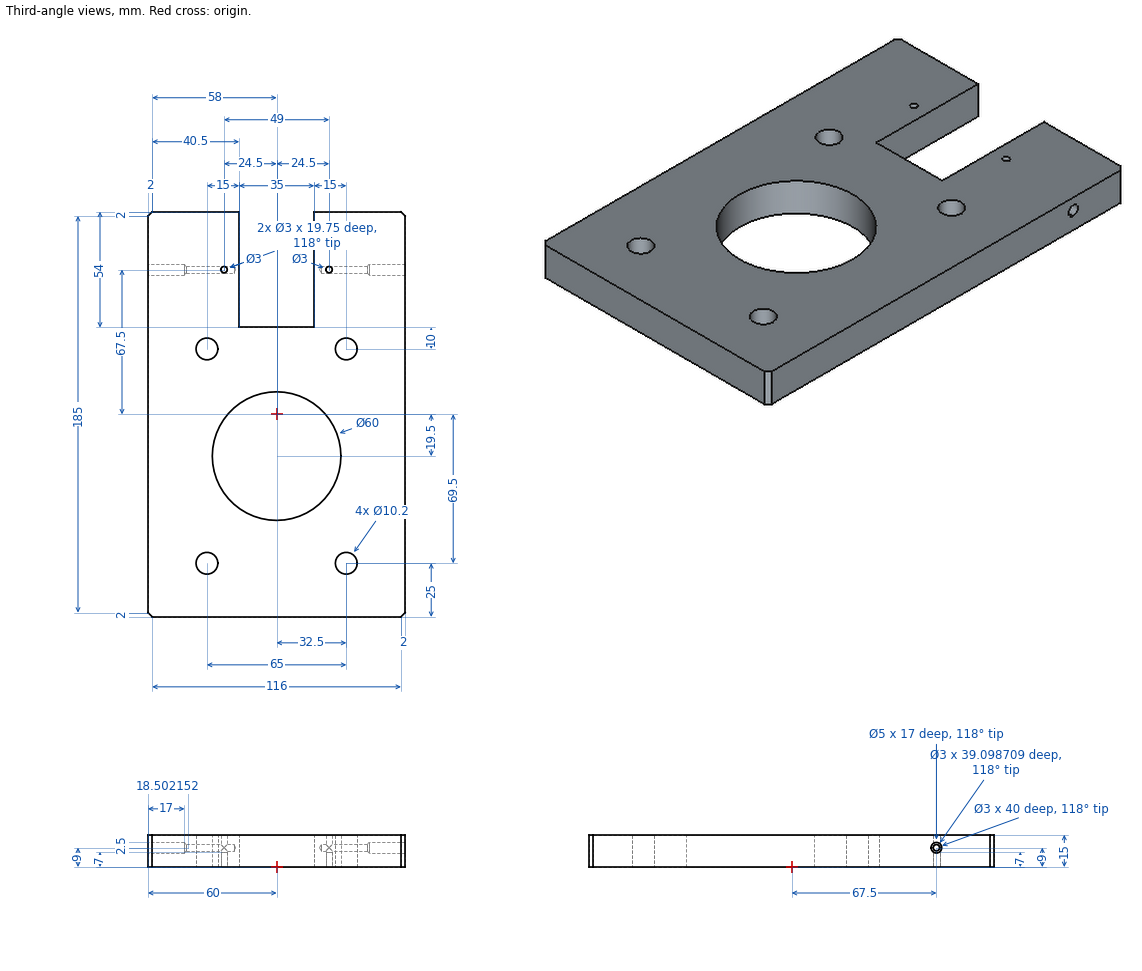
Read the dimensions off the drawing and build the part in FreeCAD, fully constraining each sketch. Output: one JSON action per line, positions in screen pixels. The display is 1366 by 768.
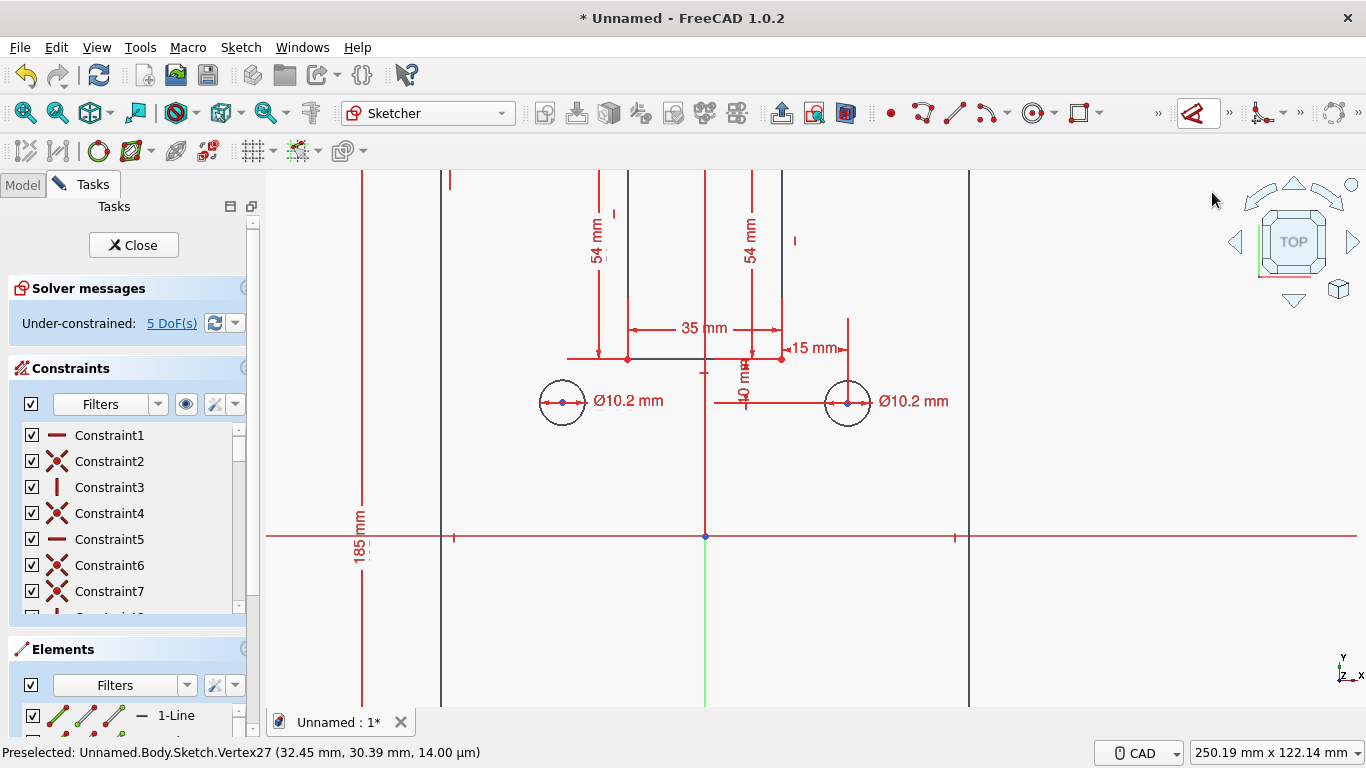
{"action": "left_click", "coordinate": [628, 359]}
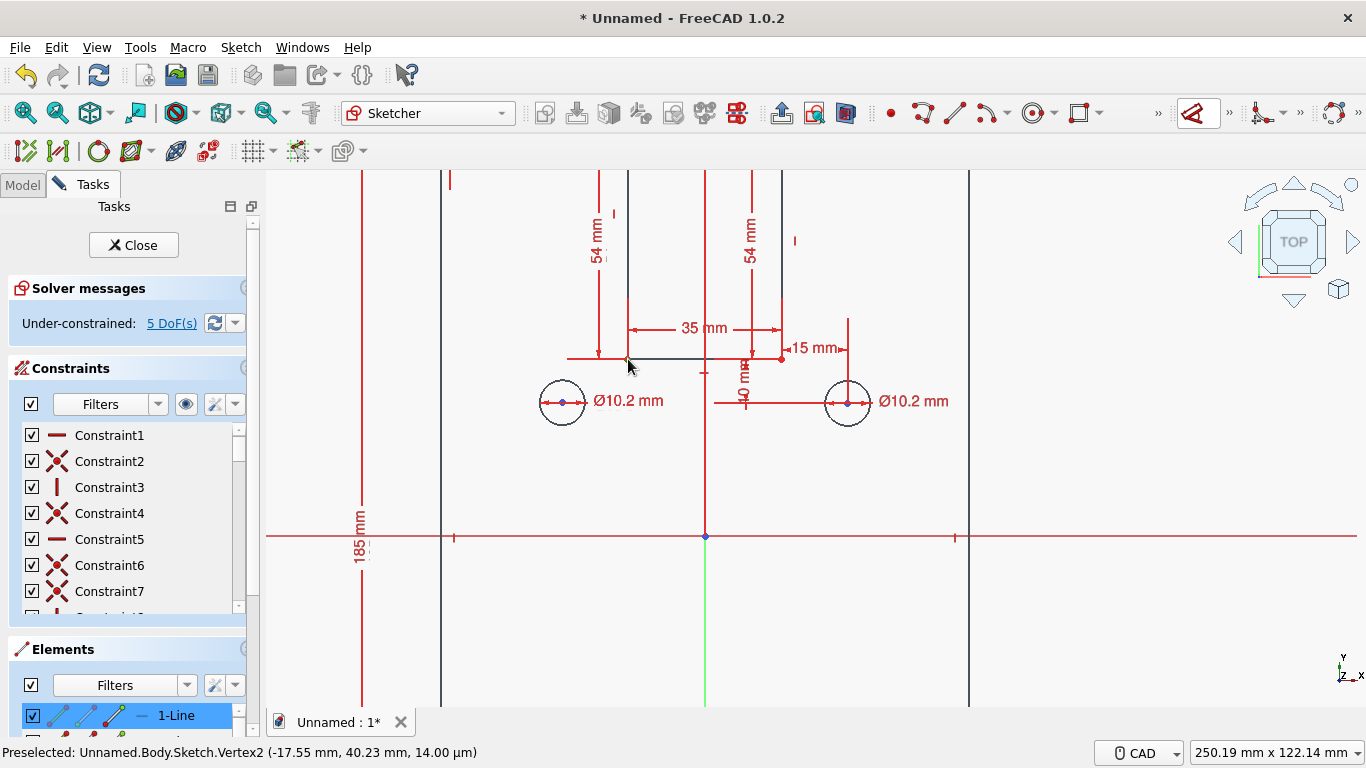
{"action": "left_click", "coordinate": [562, 403]}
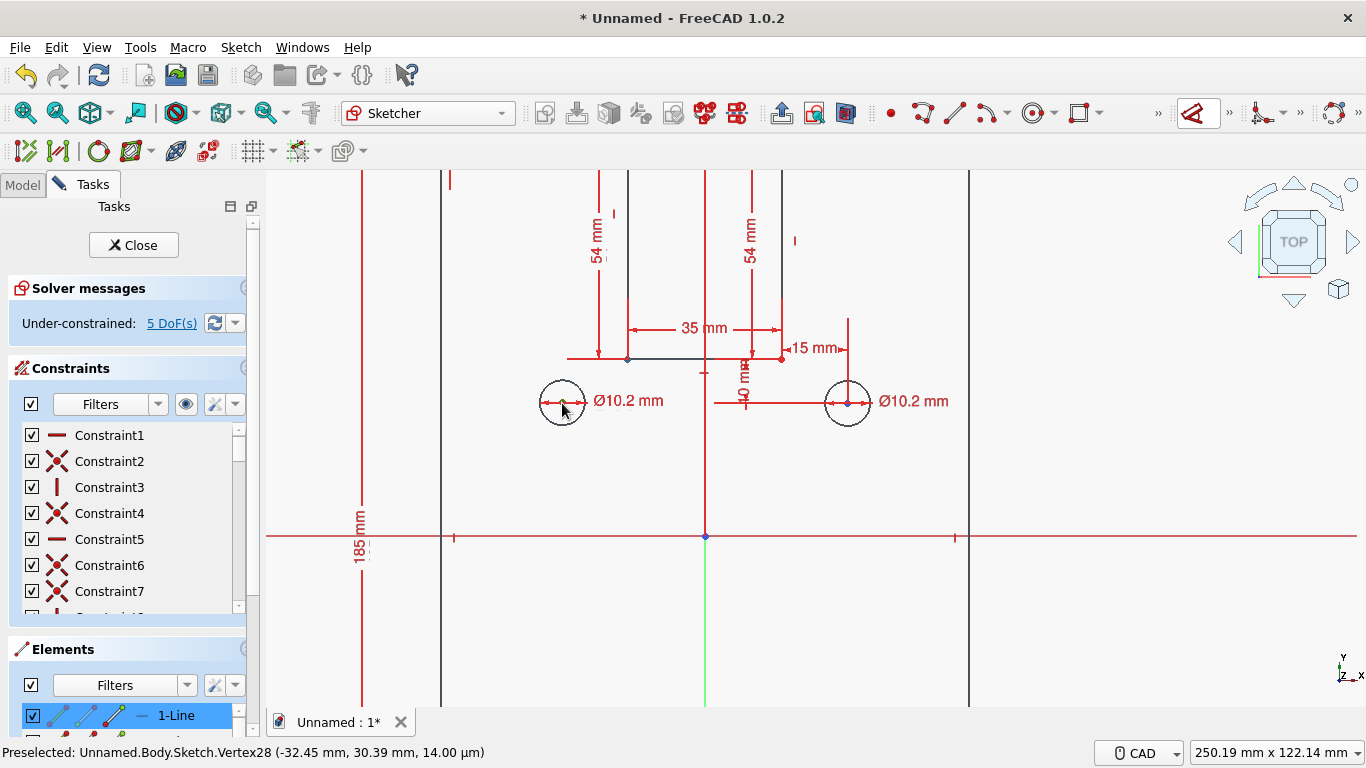
{"action": "key", "text": "l"}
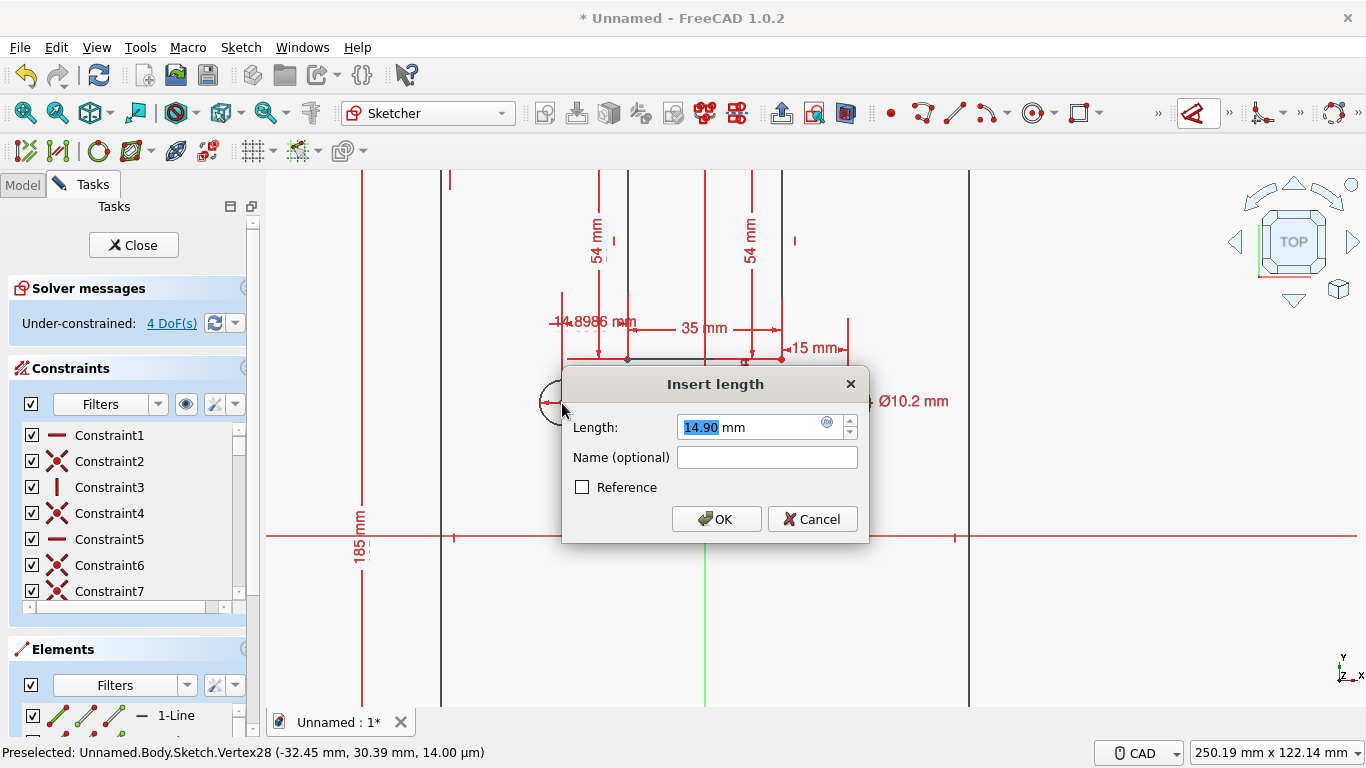
{"action": "type", "text": "15"}
{"action": "key", "text": "Return"}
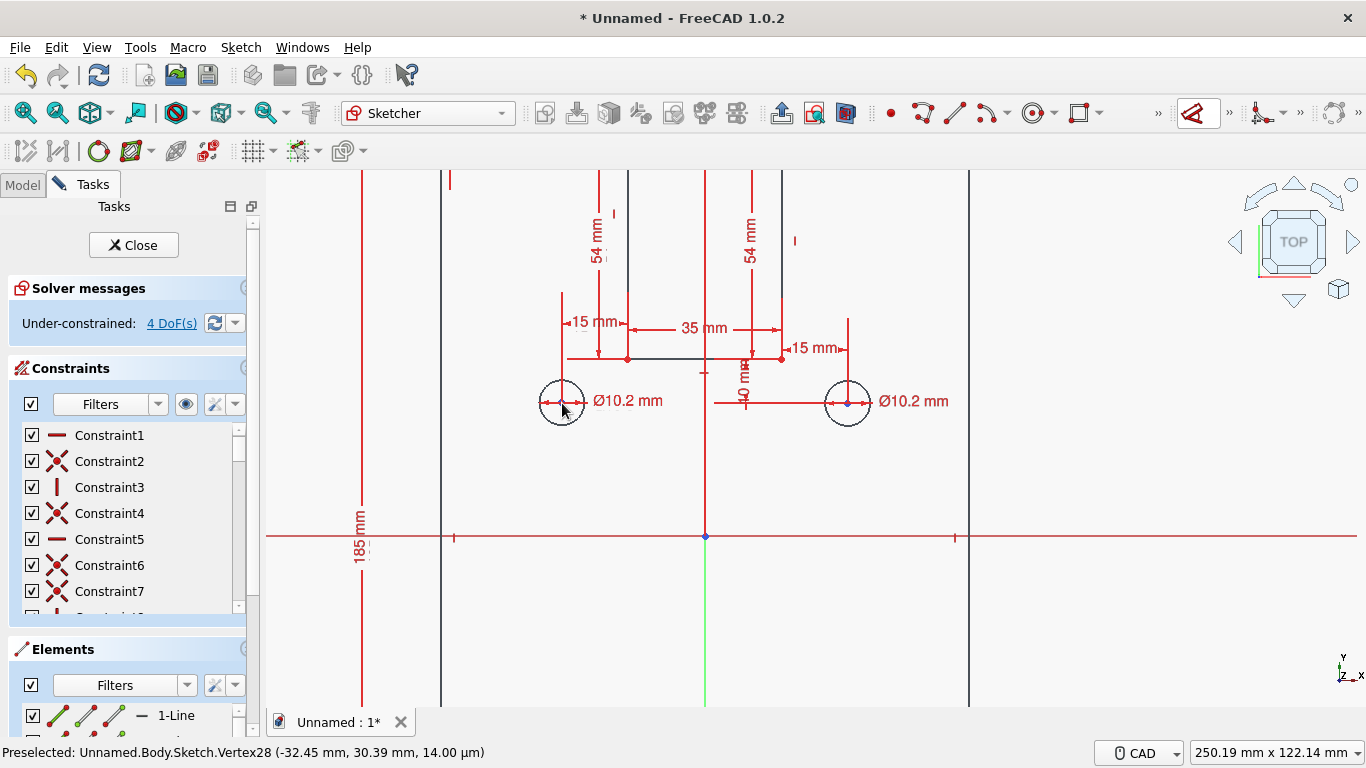
{"action": "left_click", "coordinate": [628, 359]}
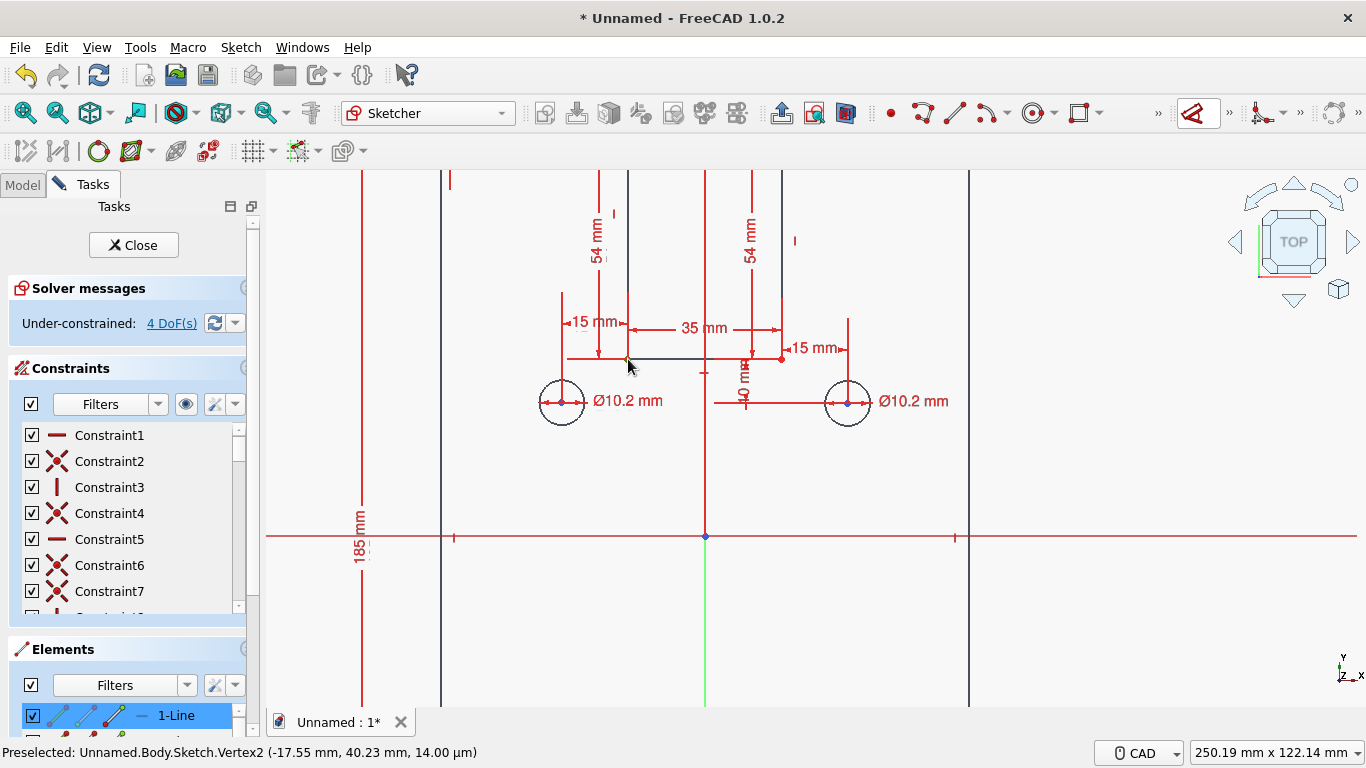
{"action": "left_click", "coordinate": [562, 403]}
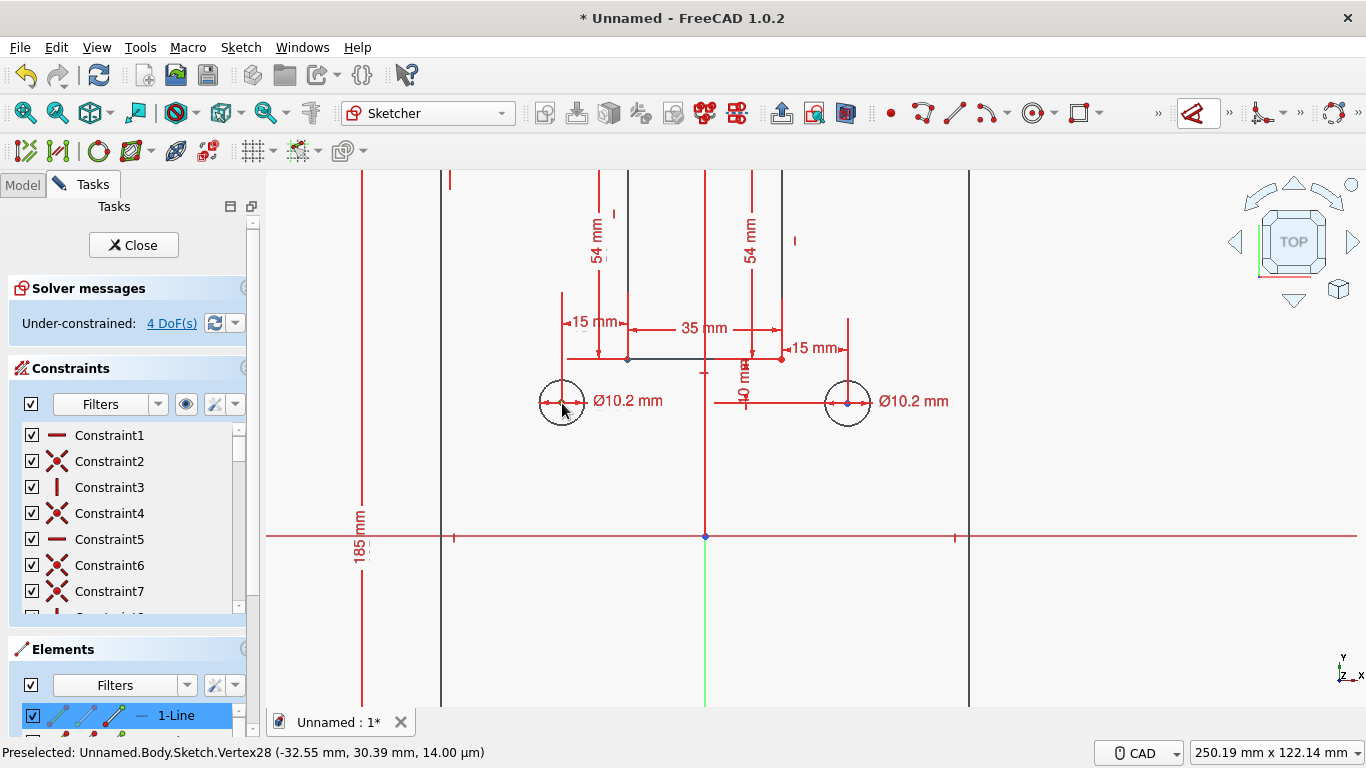
{"action": "key", "text": "i"}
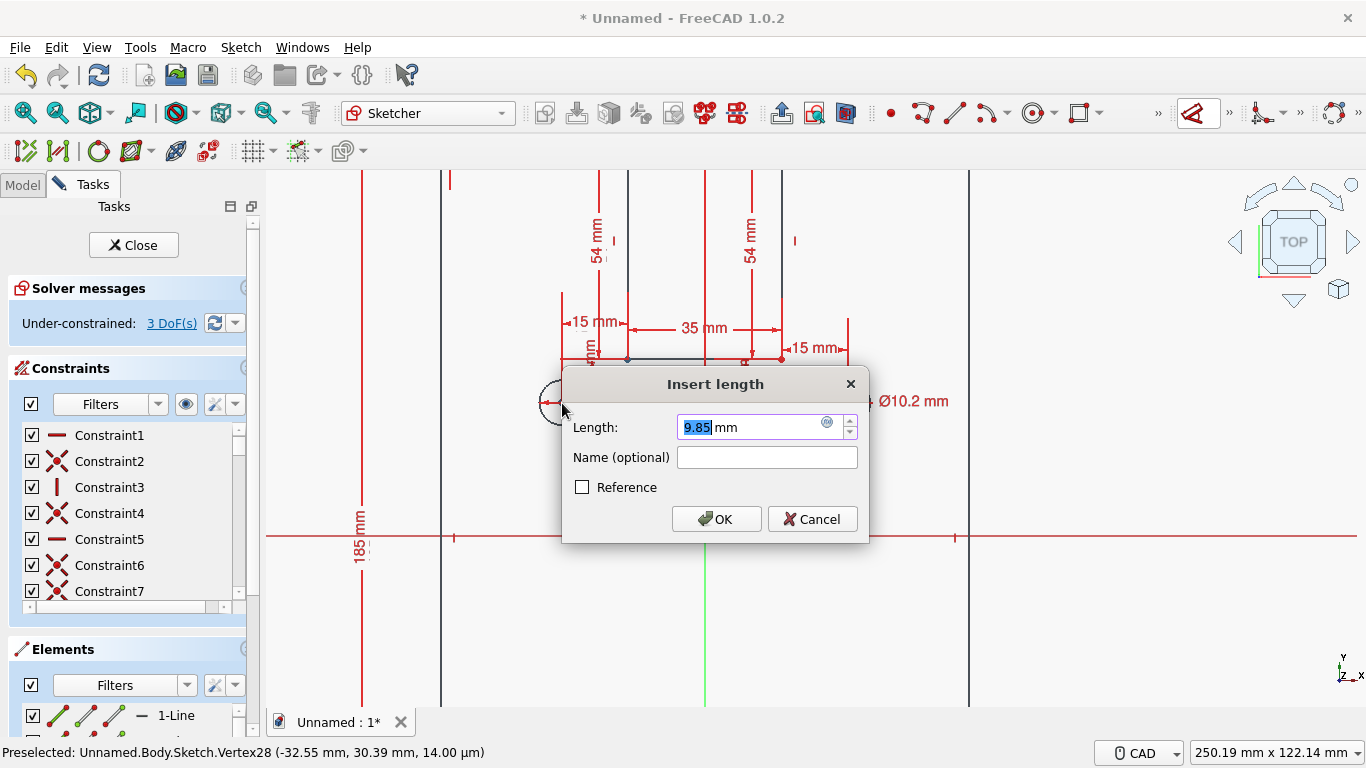
{"action": "type", "text": "10"}
{"action": "key", "text": "Return"}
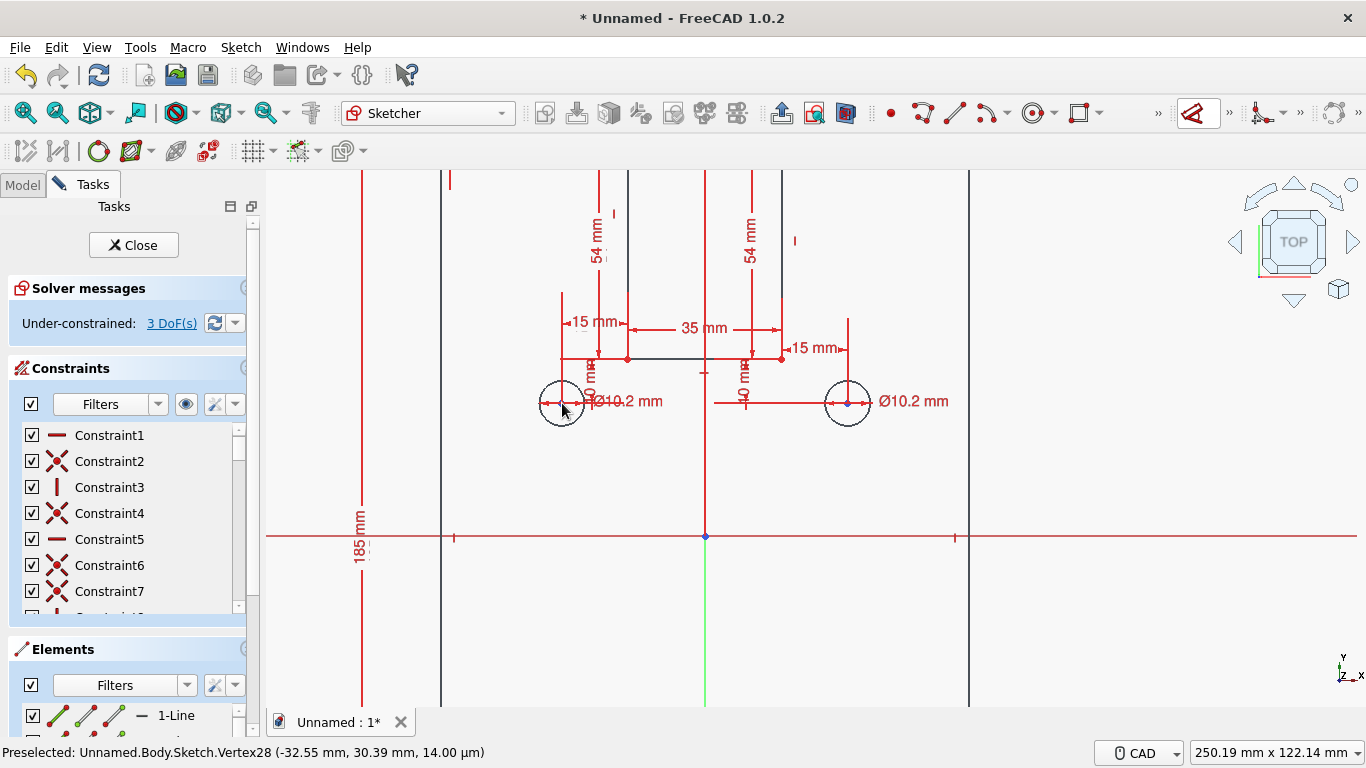
{"action": "scroll", "coordinate": [782, 359], "scroll_direction": "down", "scroll_amount": 4}